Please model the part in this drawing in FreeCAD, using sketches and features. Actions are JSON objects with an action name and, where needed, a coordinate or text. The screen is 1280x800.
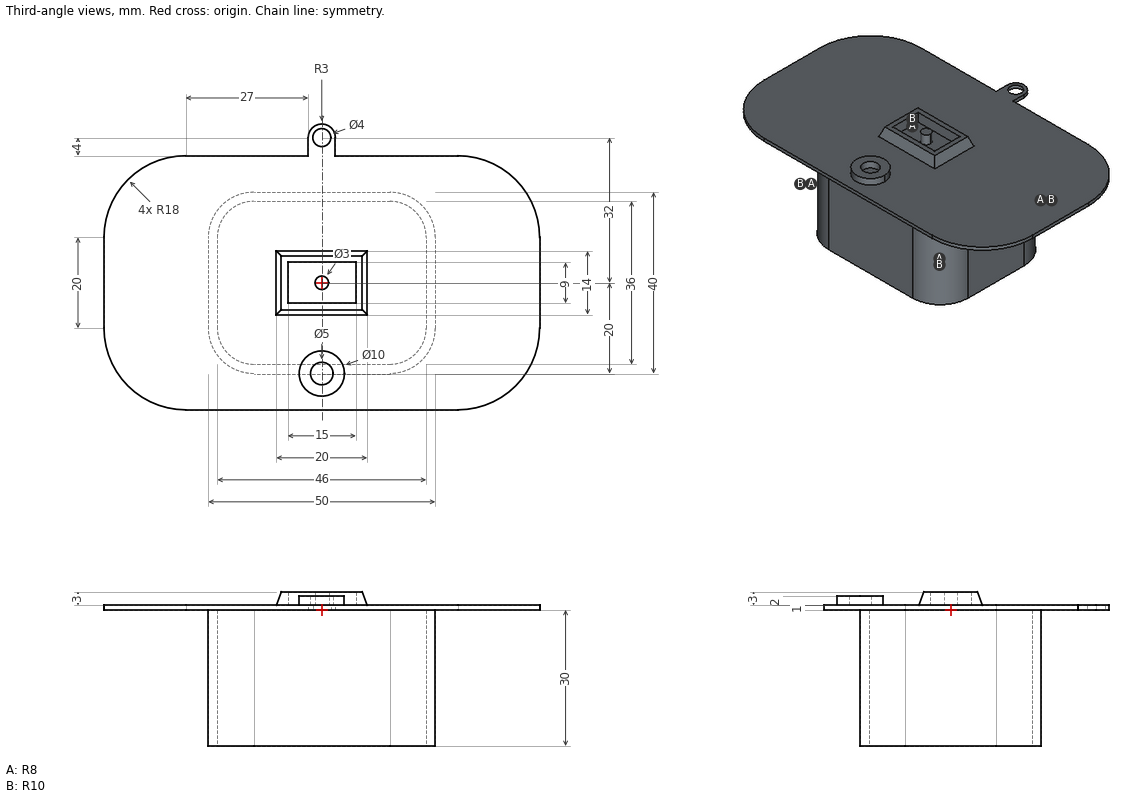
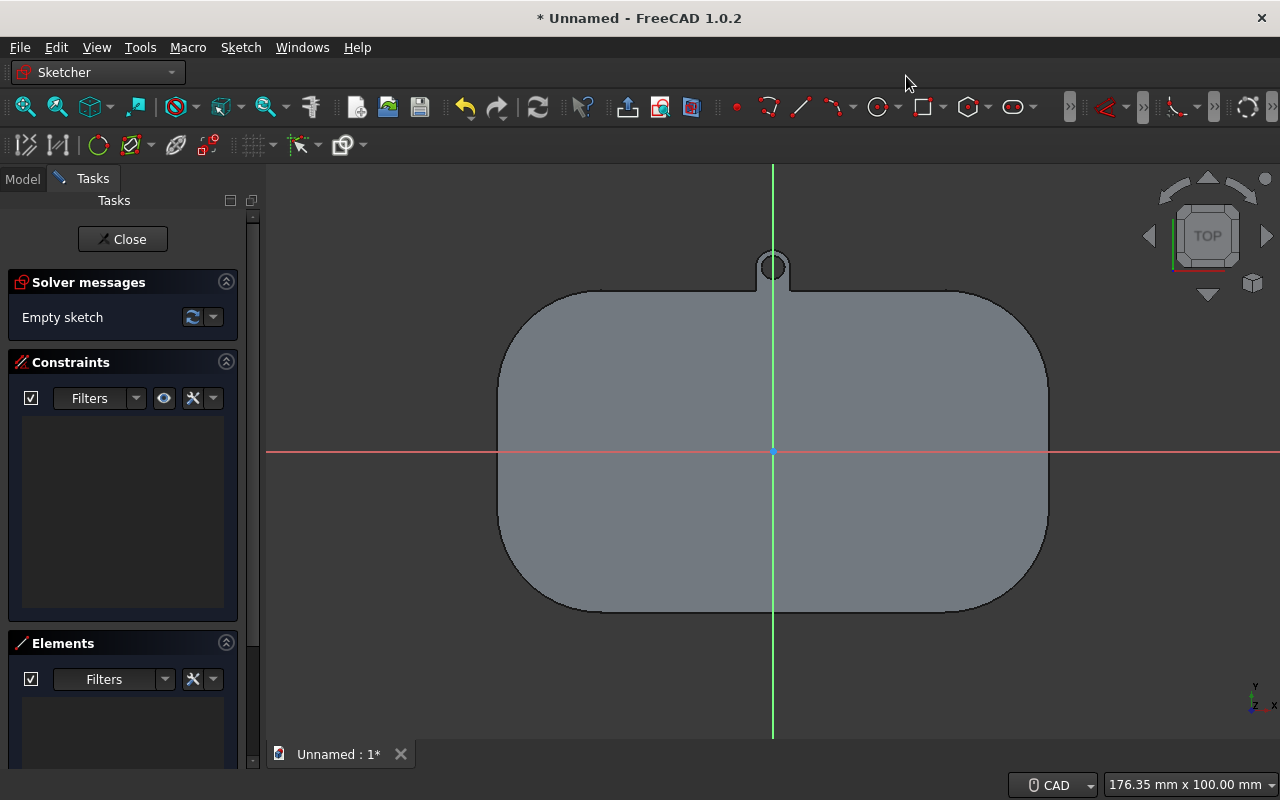
{"action": "scroll", "coordinate": [790, 451], "scroll_direction": "up", "scroll_amount": 8}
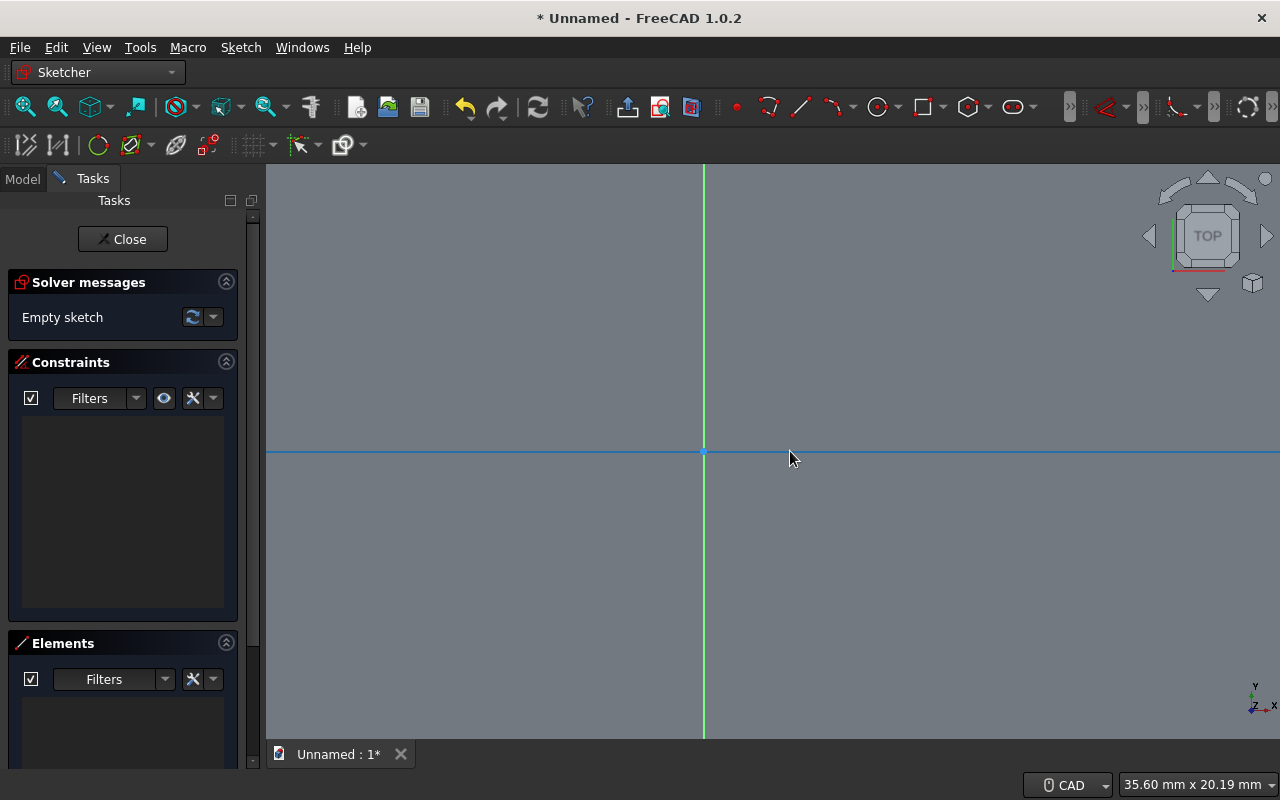
{"action": "left_click", "coordinate": [946, 108]}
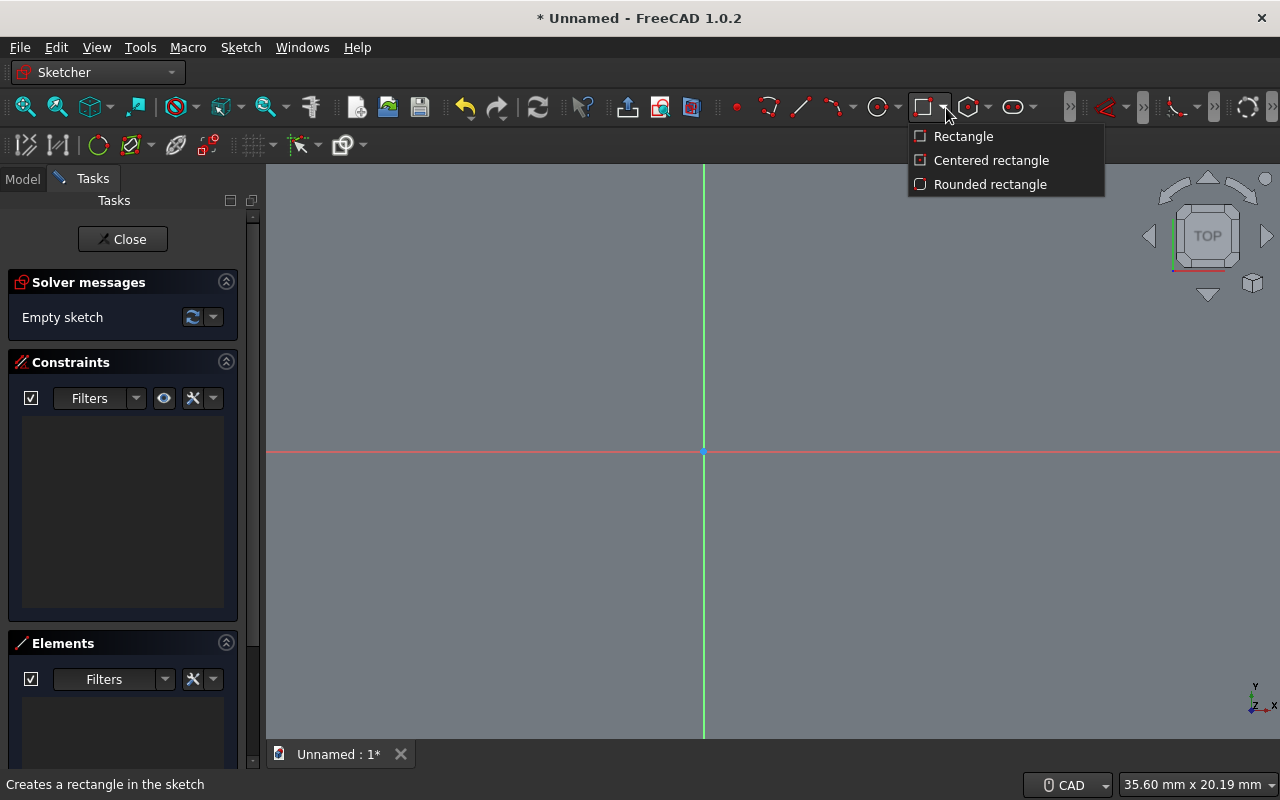
{"action": "left_click", "coordinate": [1006, 160]}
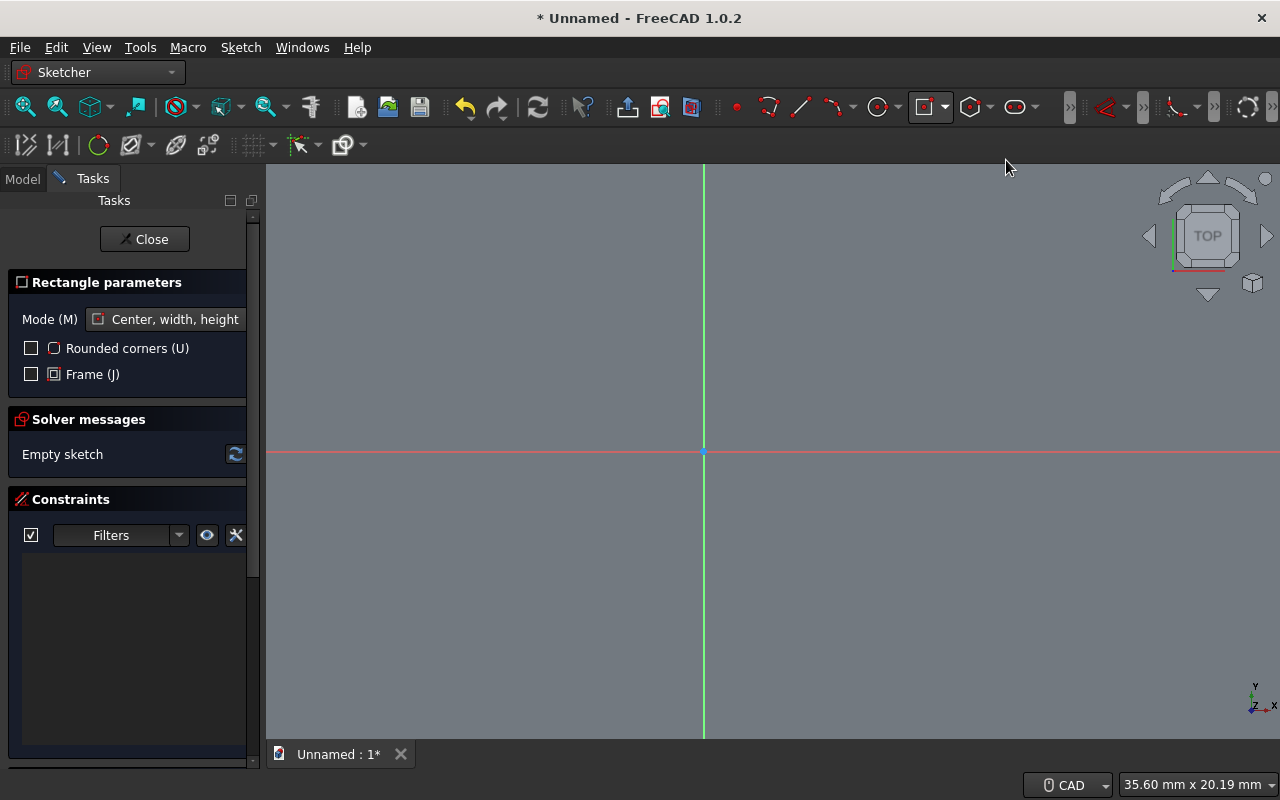
{"action": "left_click", "coordinate": [704, 452]}
{"action": "mouse_move", "coordinate": [989, 252]}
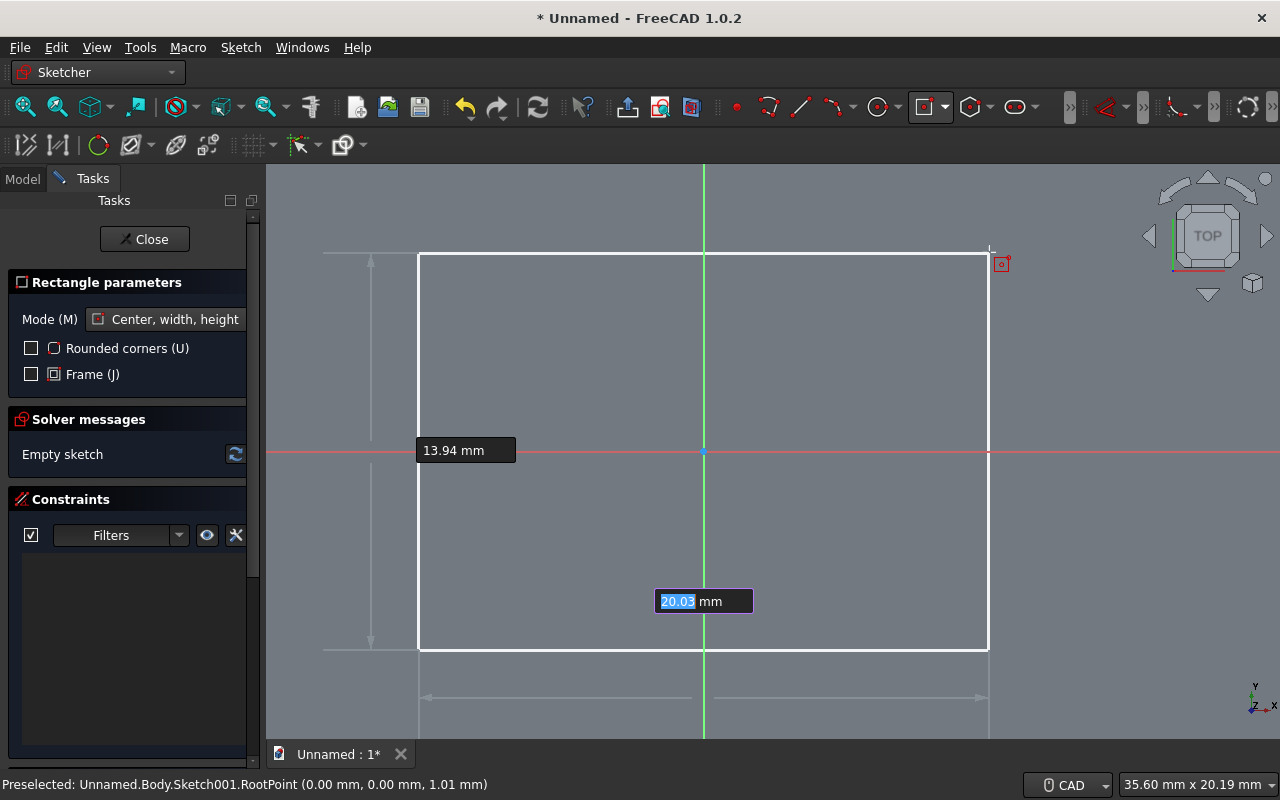
{"action": "type", "text": "20"}
{"action": "key", "text": "Tab"}
{"action": "type", "text": "14"}
{"action": "key", "text": "Return"}
{"action": "key", "text": "Escape"}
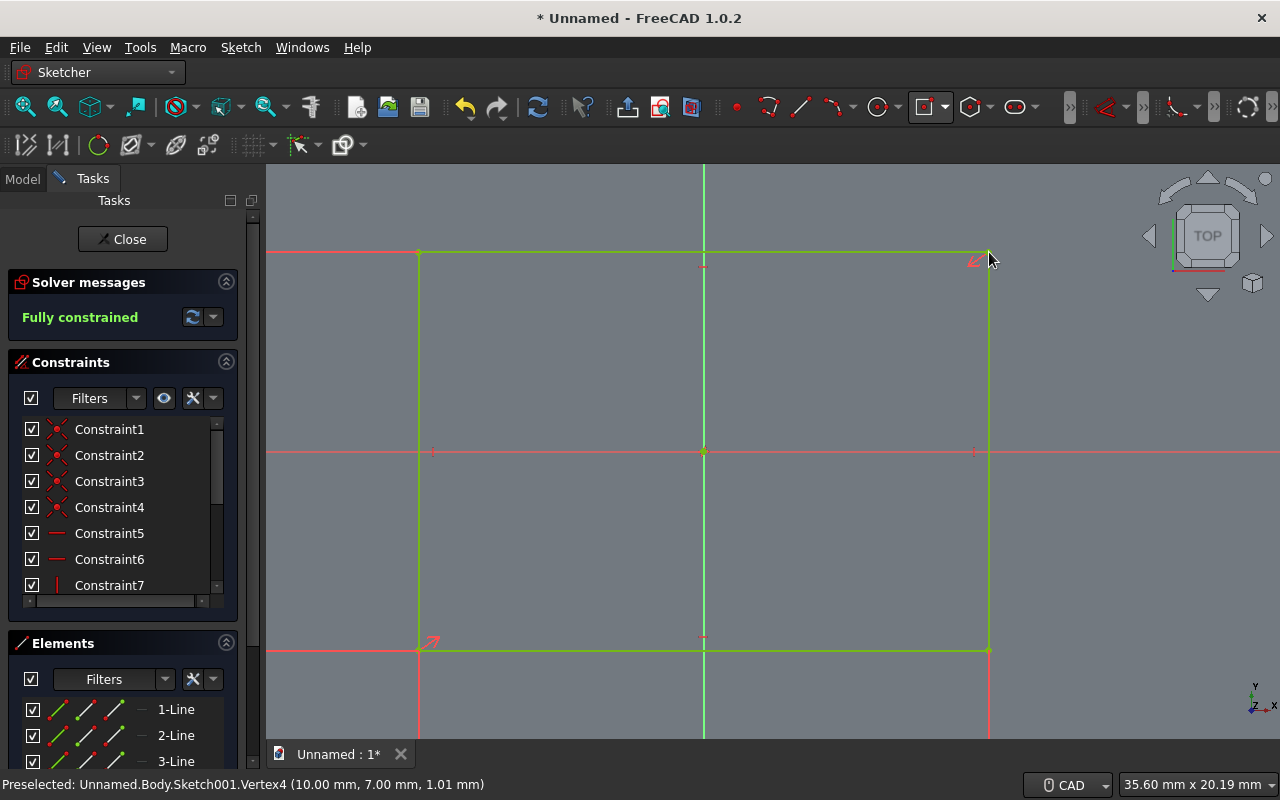
{"action": "left_click", "coordinate": [123, 239]}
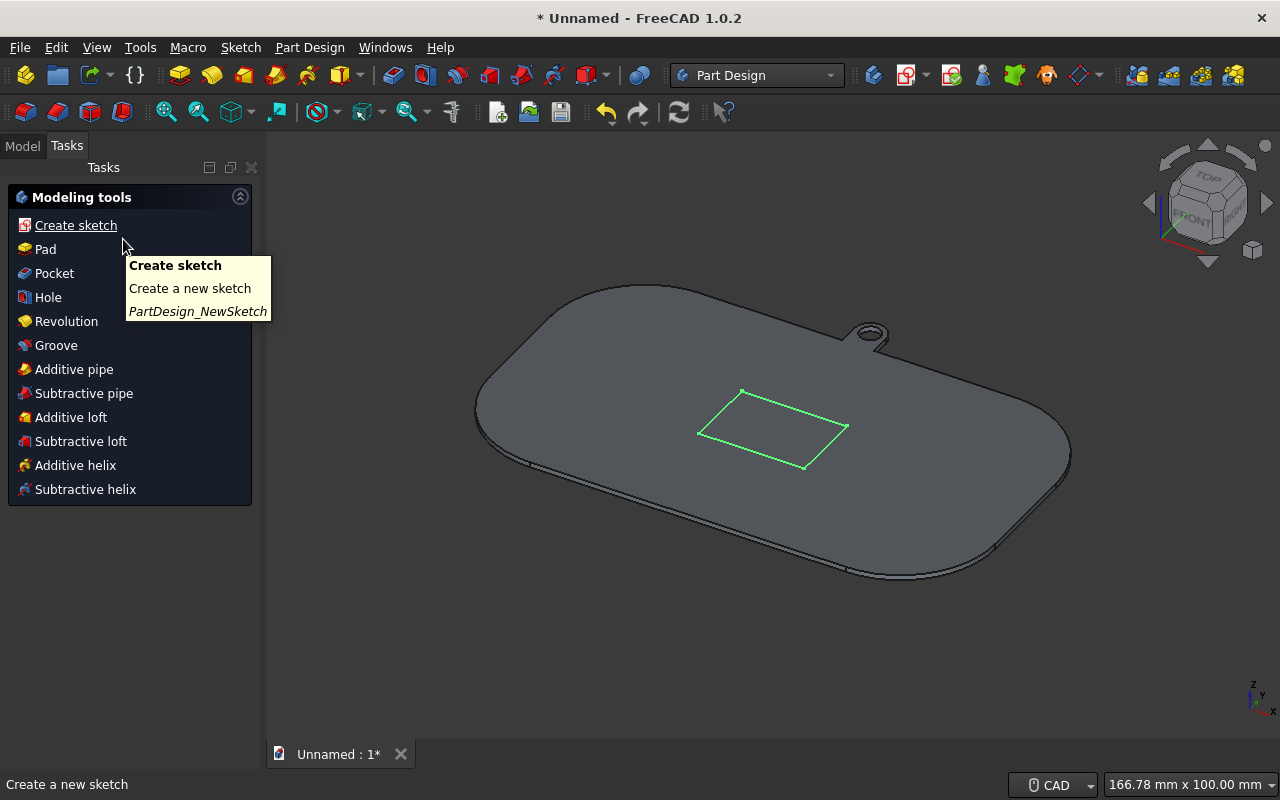
{"action": "left_click", "coordinate": [180, 76]}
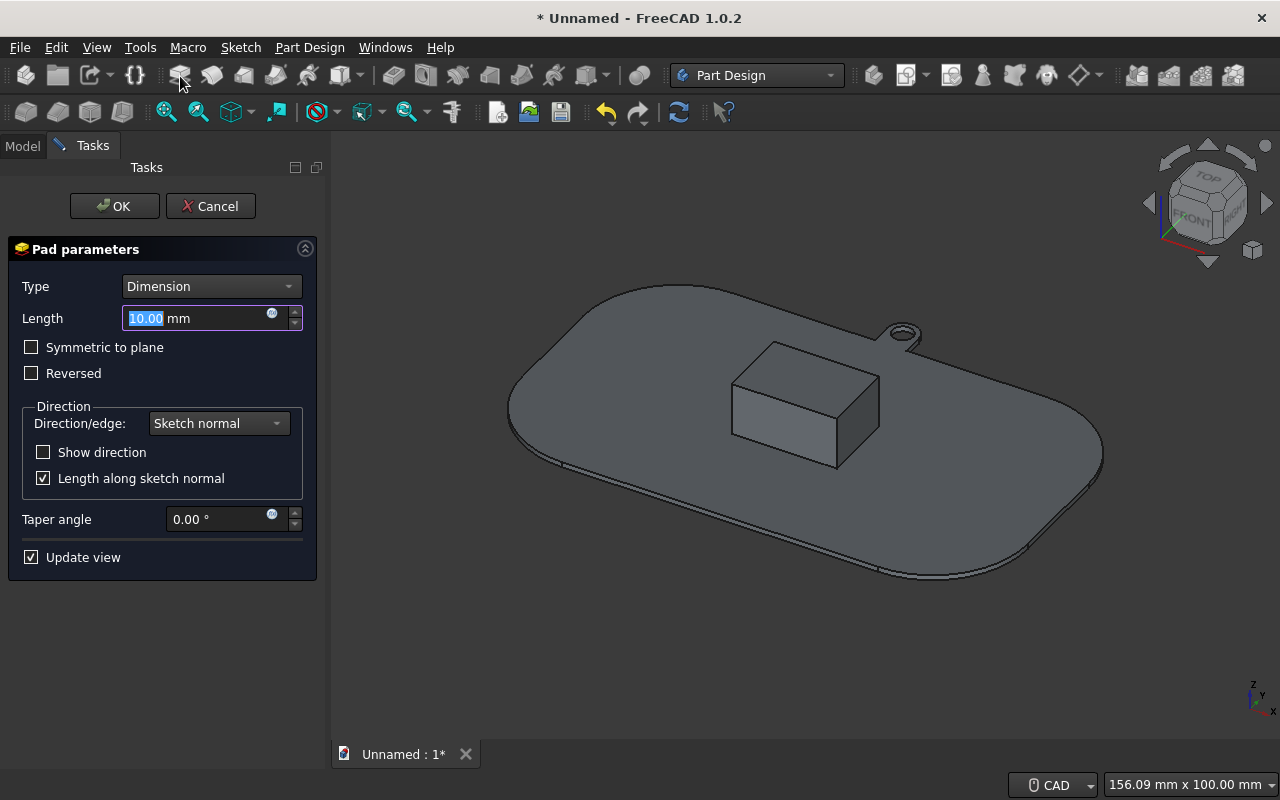
{"action": "type", "text": "3"}
{"action": "key", "text": "Tab"}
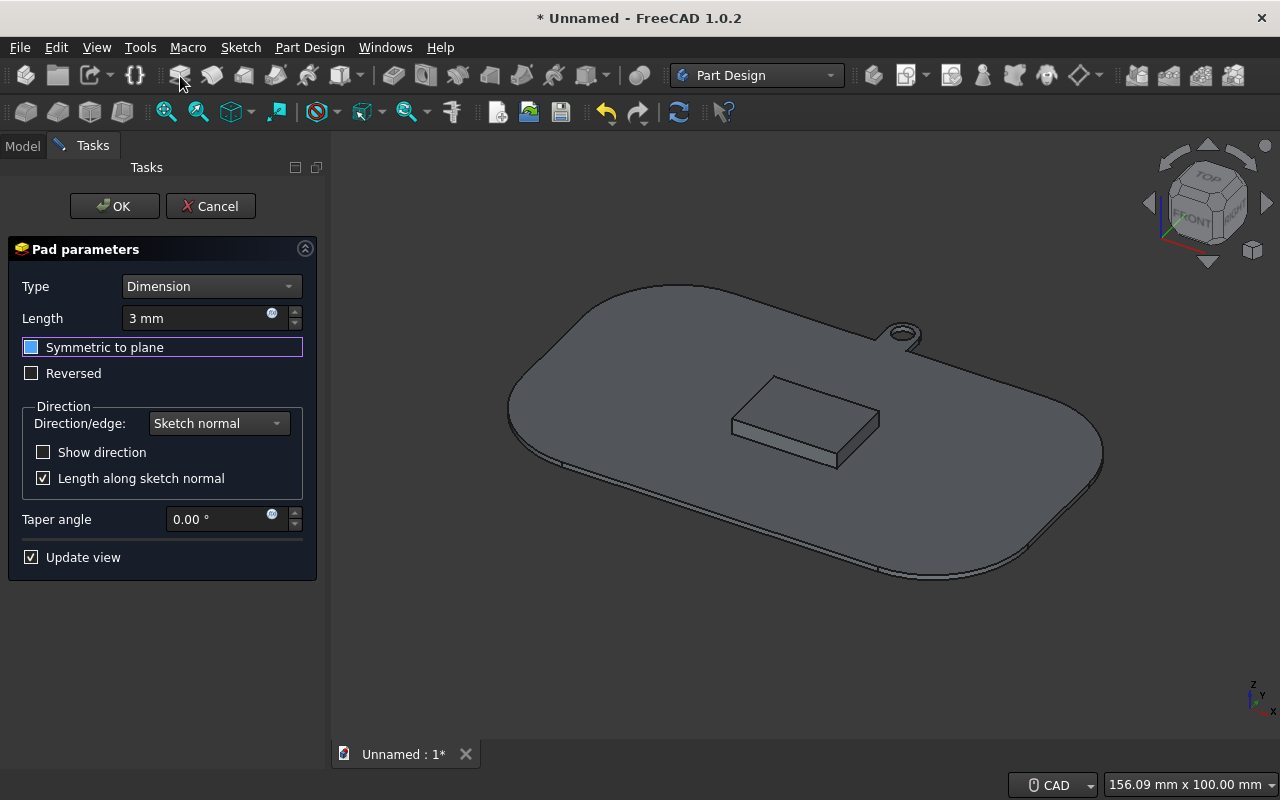
{"action": "triple_click", "coordinate": [226, 519]}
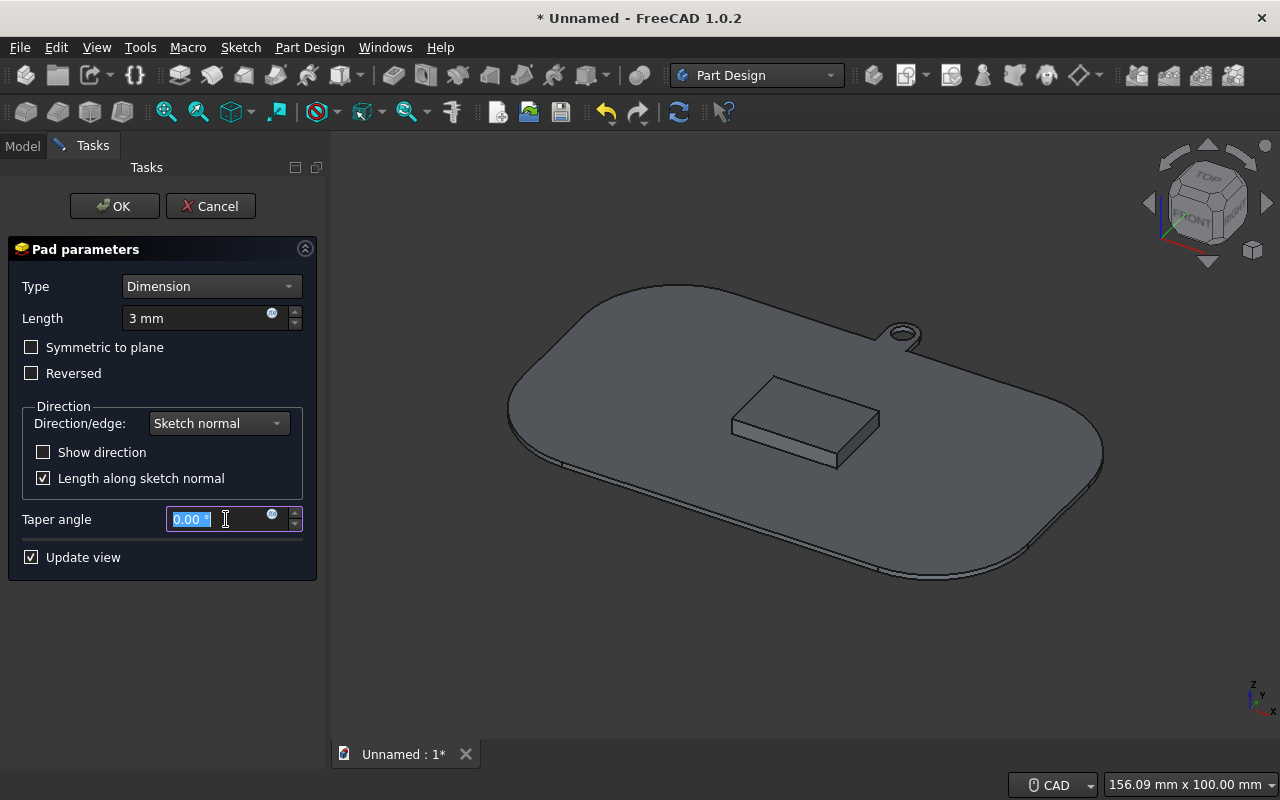
{"action": "type", "text": "-20"}
{"action": "key", "text": "Tab"}